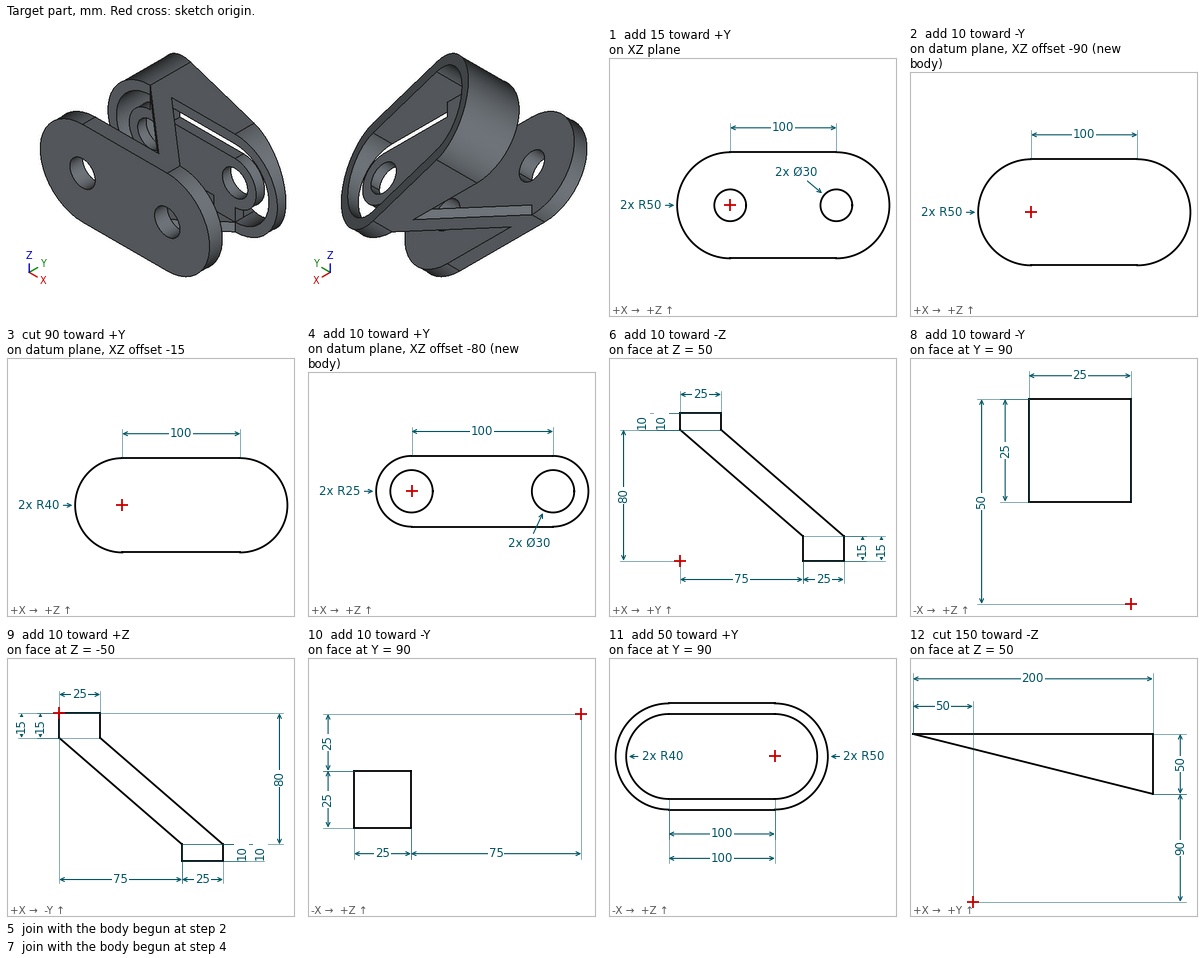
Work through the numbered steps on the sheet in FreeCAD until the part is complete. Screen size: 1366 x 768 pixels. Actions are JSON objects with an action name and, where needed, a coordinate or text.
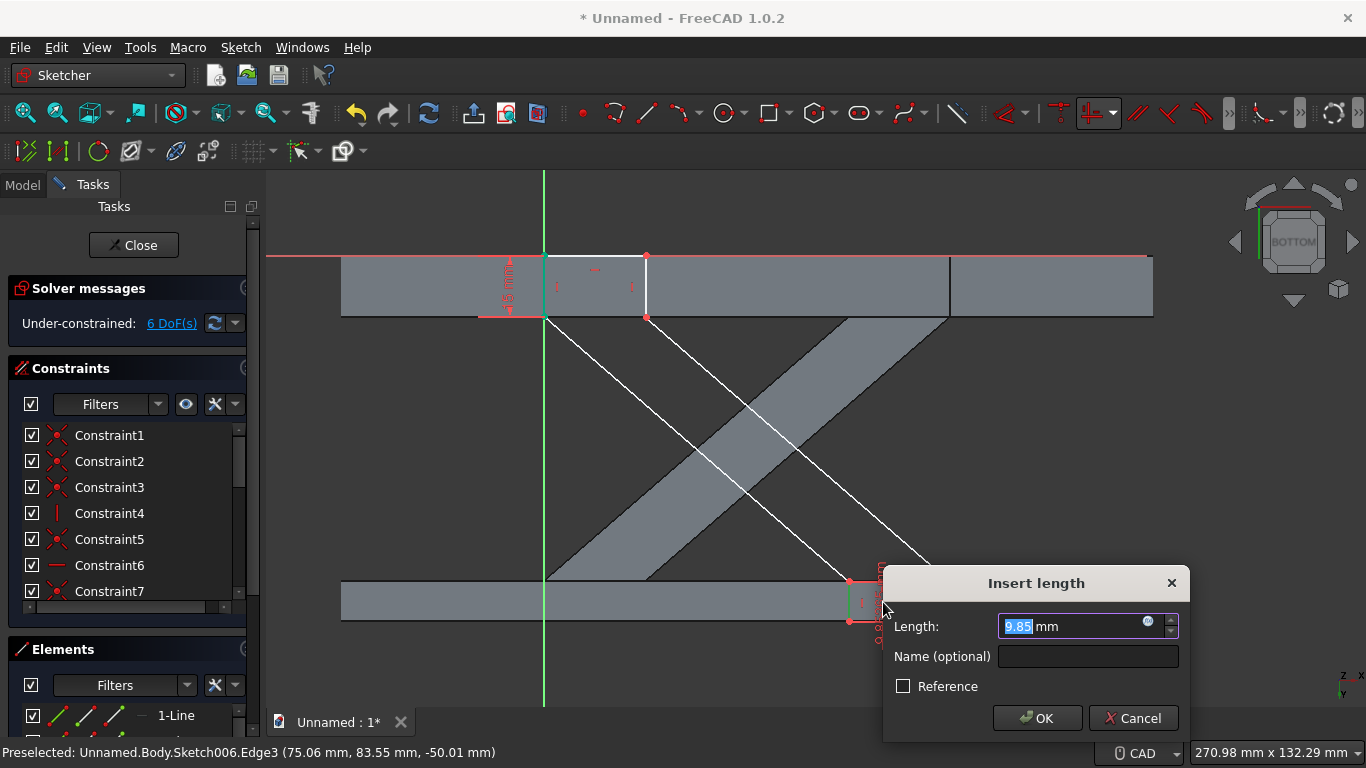
{"action": "type", "text": "10"}
{"action": "key", "text": "Return"}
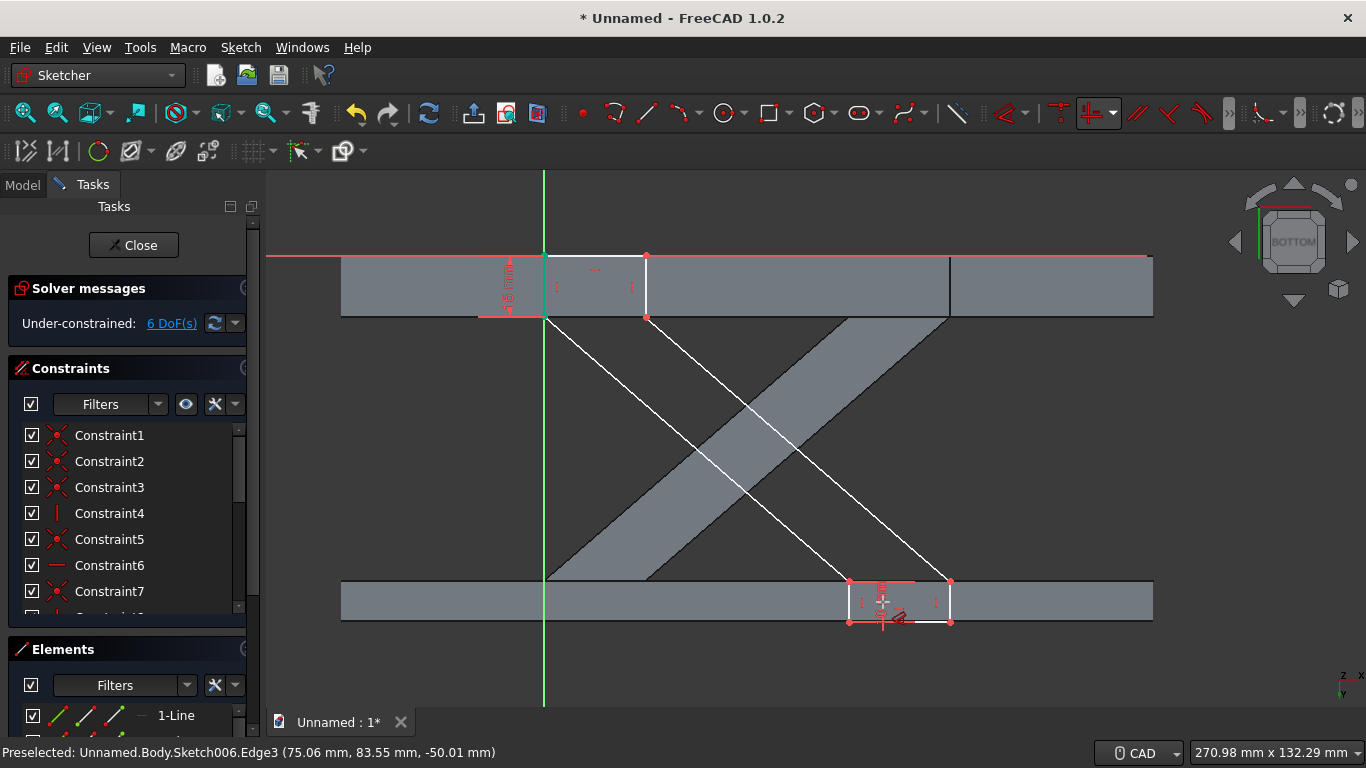
{"action": "left_click", "coordinate": [879, 622]}
{"action": "left_click", "coordinate": [899, 656]}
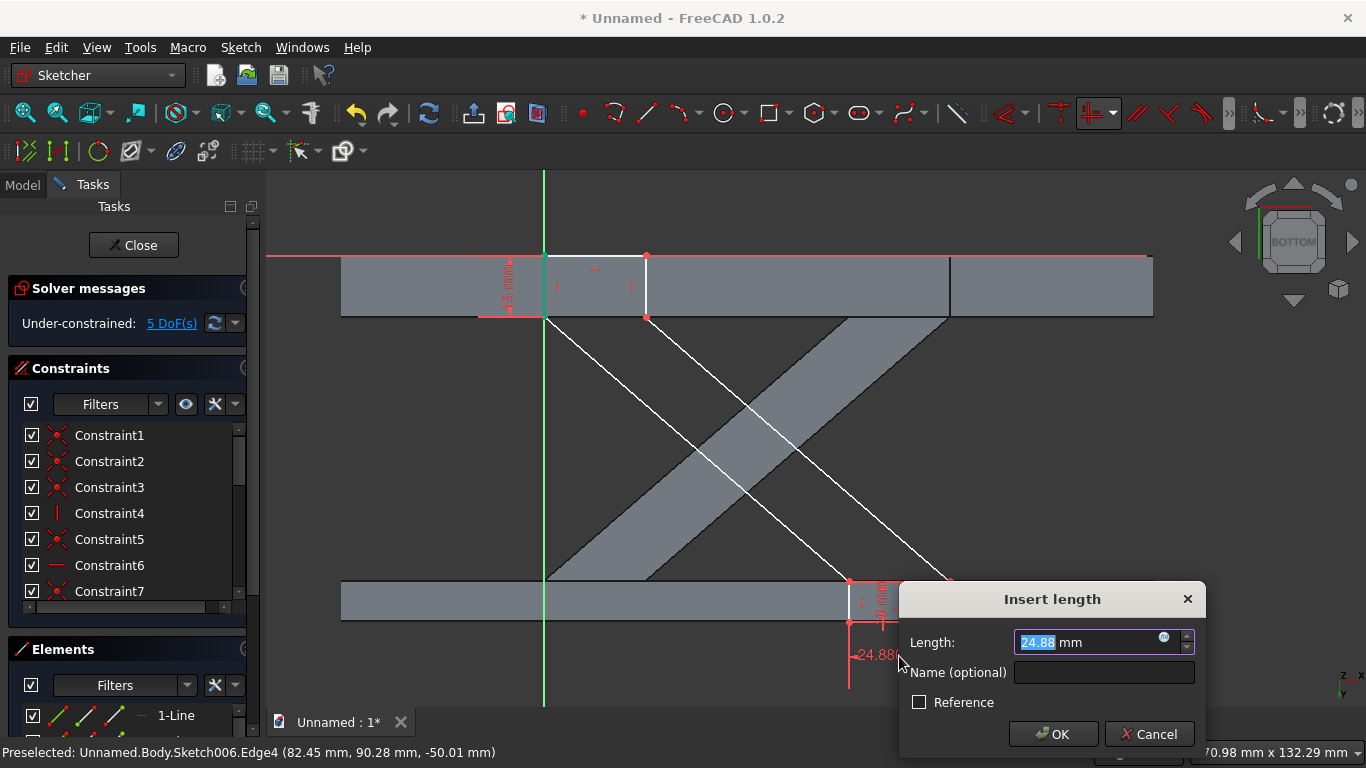
{"action": "type", "text": "25"}
{"action": "key", "text": "Return"}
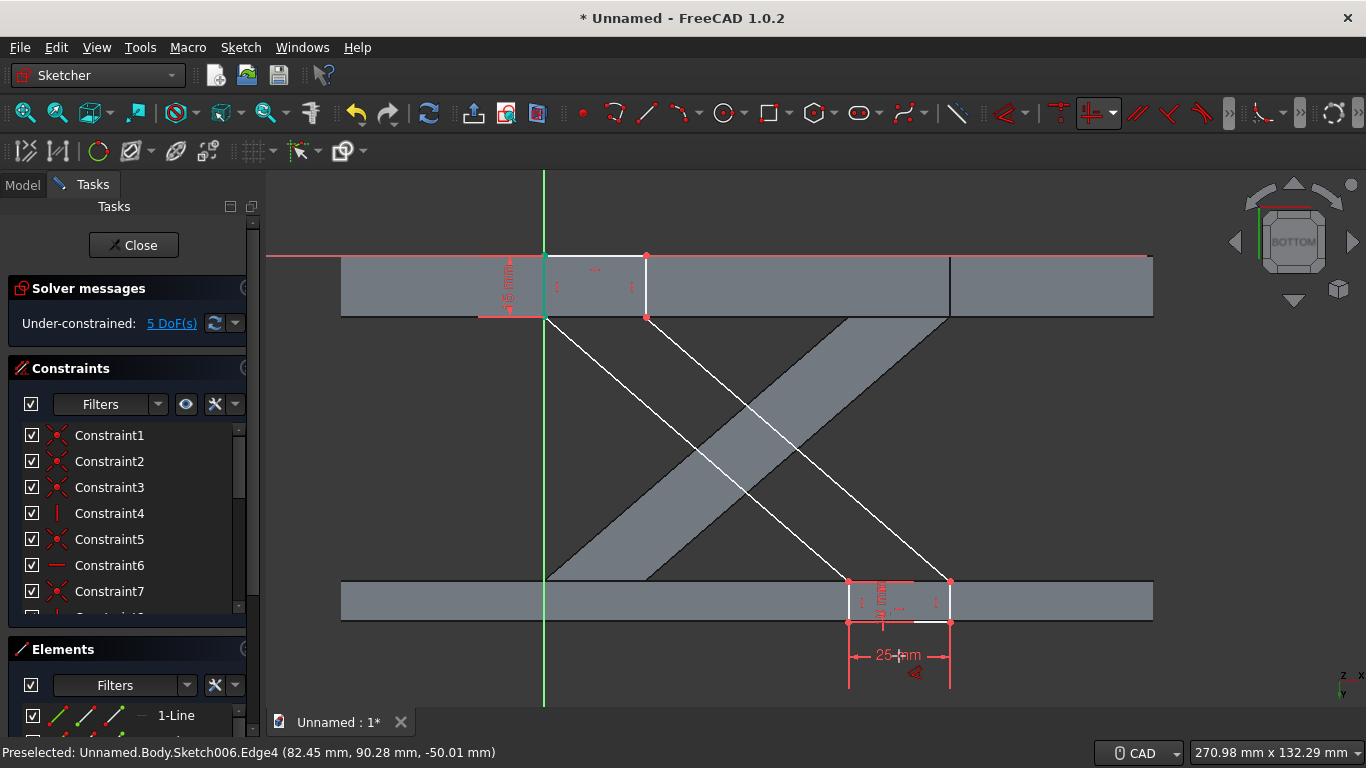
{"action": "left_click", "coordinate": [950, 610]}
{"action": "left_click", "coordinate": [984, 602]}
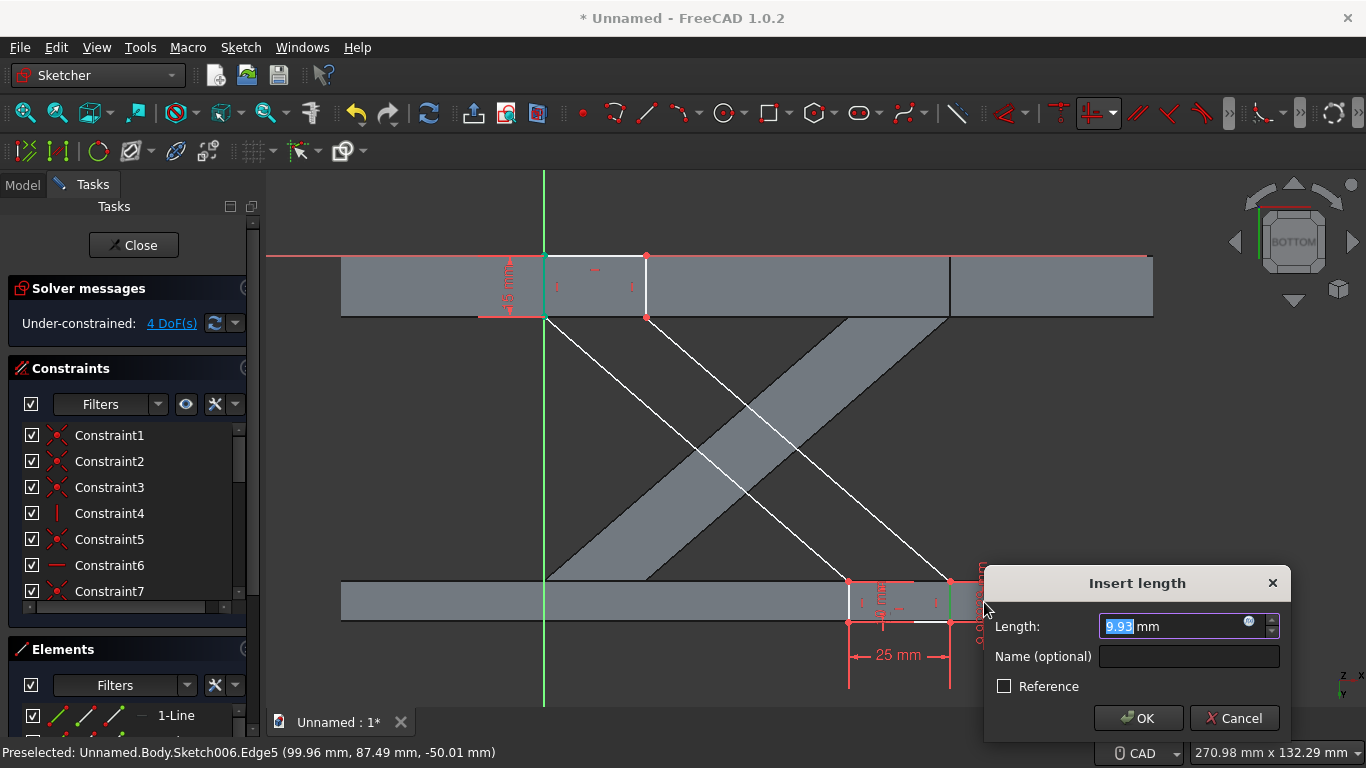
{"action": "type", "text": "10"}
{"action": "key", "text": "Return"}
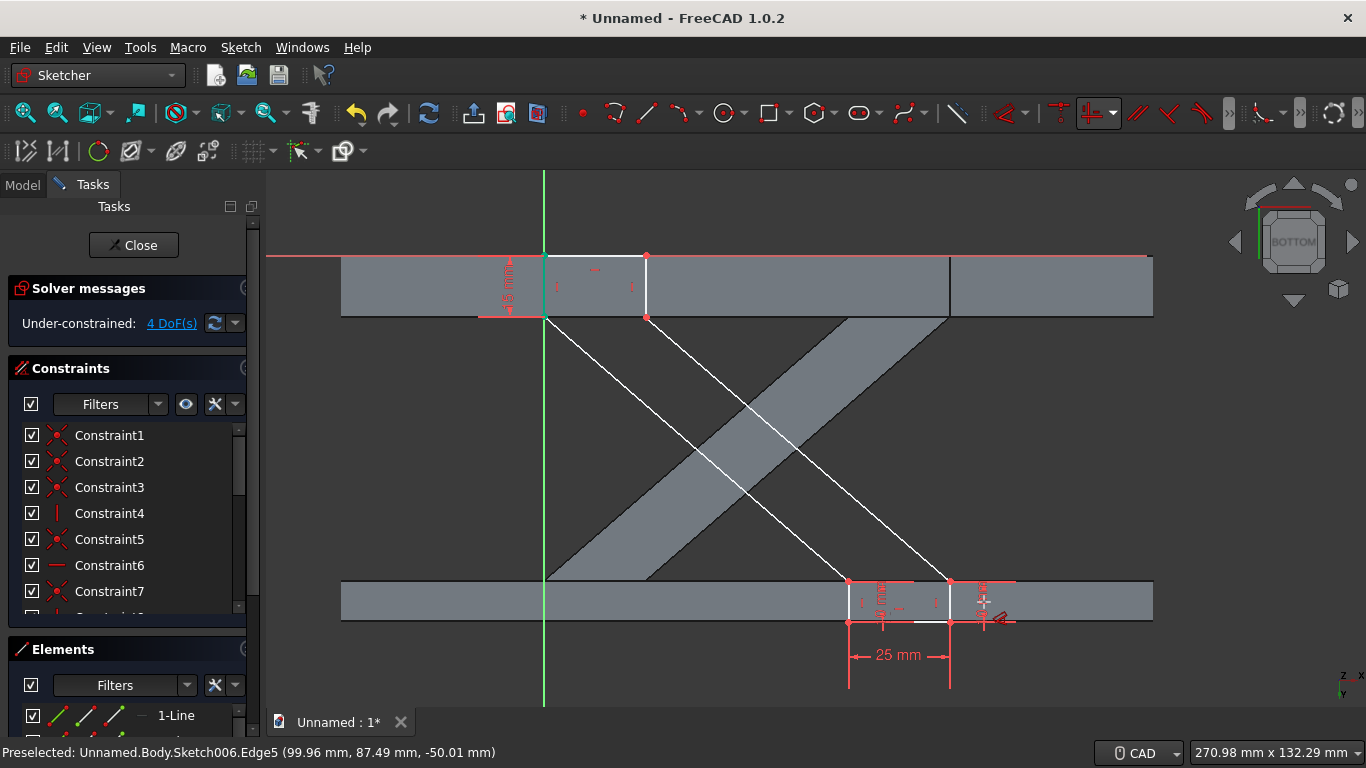
{"action": "left_click", "coordinate": [646, 299]}
{"action": "left_click", "coordinate": [612, 287]}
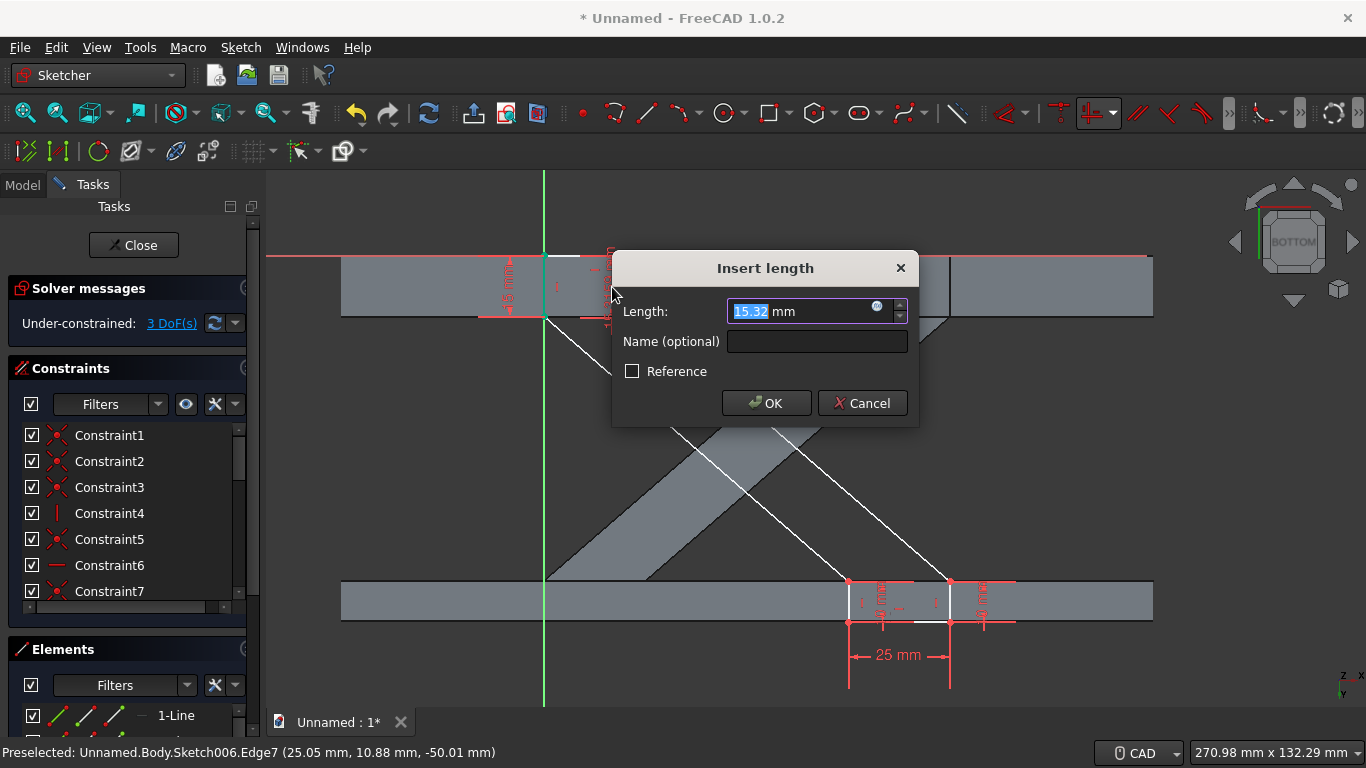
{"action": "type", "text": "15"}
{"action": "key", "text": "Return"}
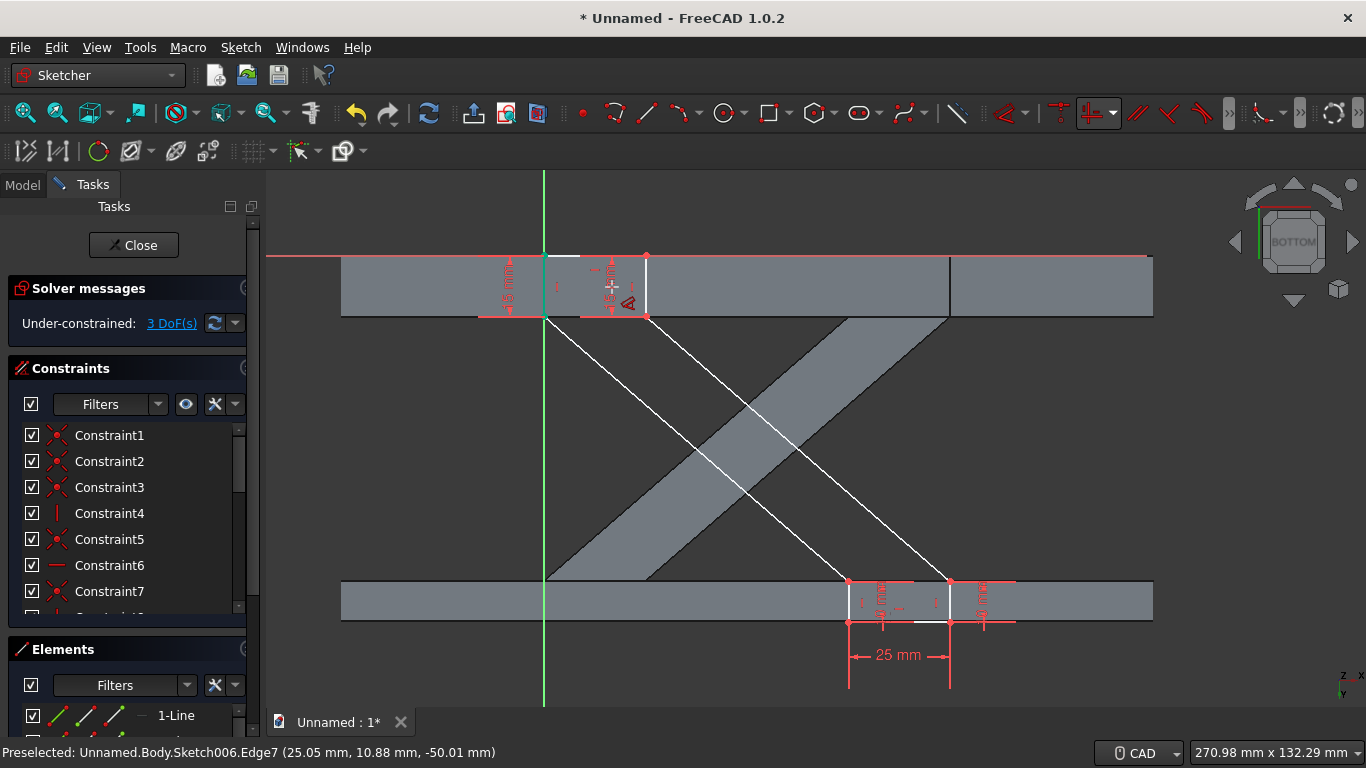
{"action": "left_click", "coordinate": [615, 256]}
{"action": "left_click", "coordinate": [595, 222]}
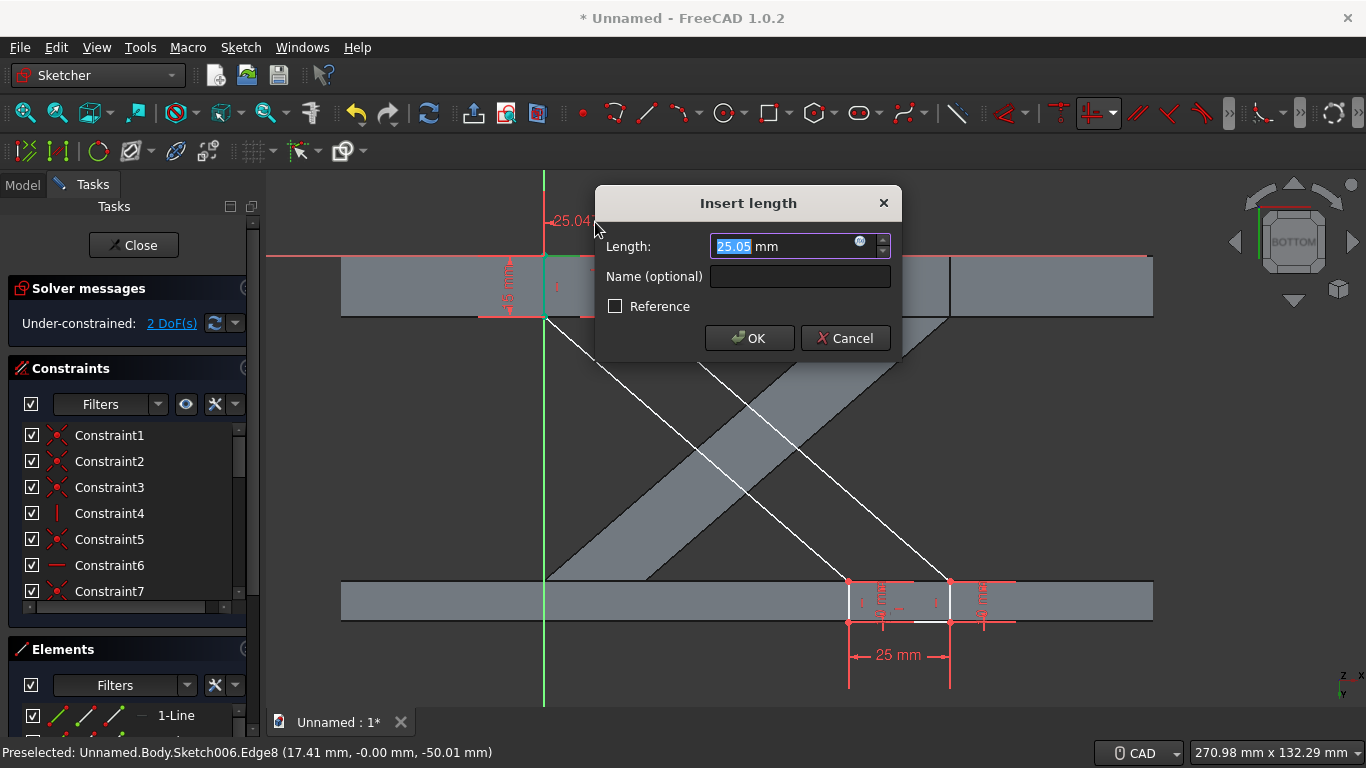
{"action": "type", "text": "25"}
{"action": "key", "text": "Return"}